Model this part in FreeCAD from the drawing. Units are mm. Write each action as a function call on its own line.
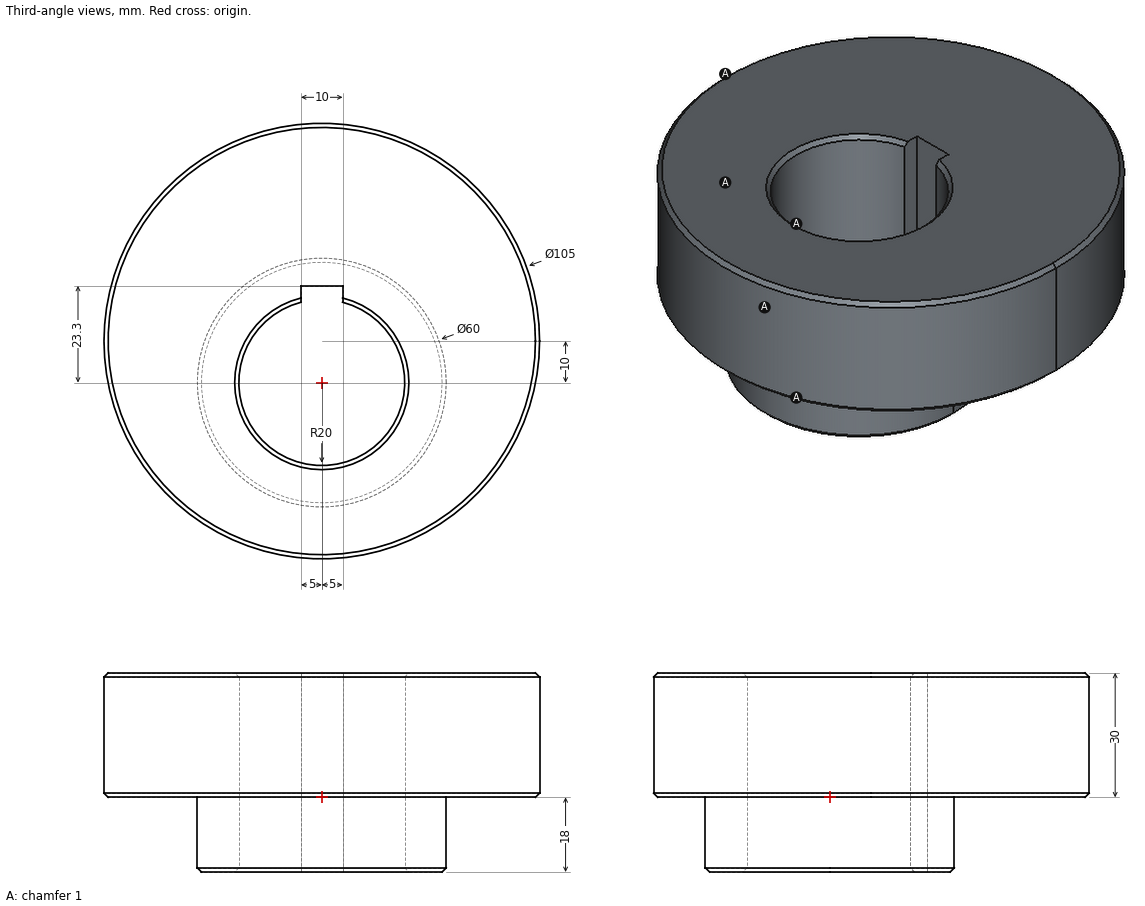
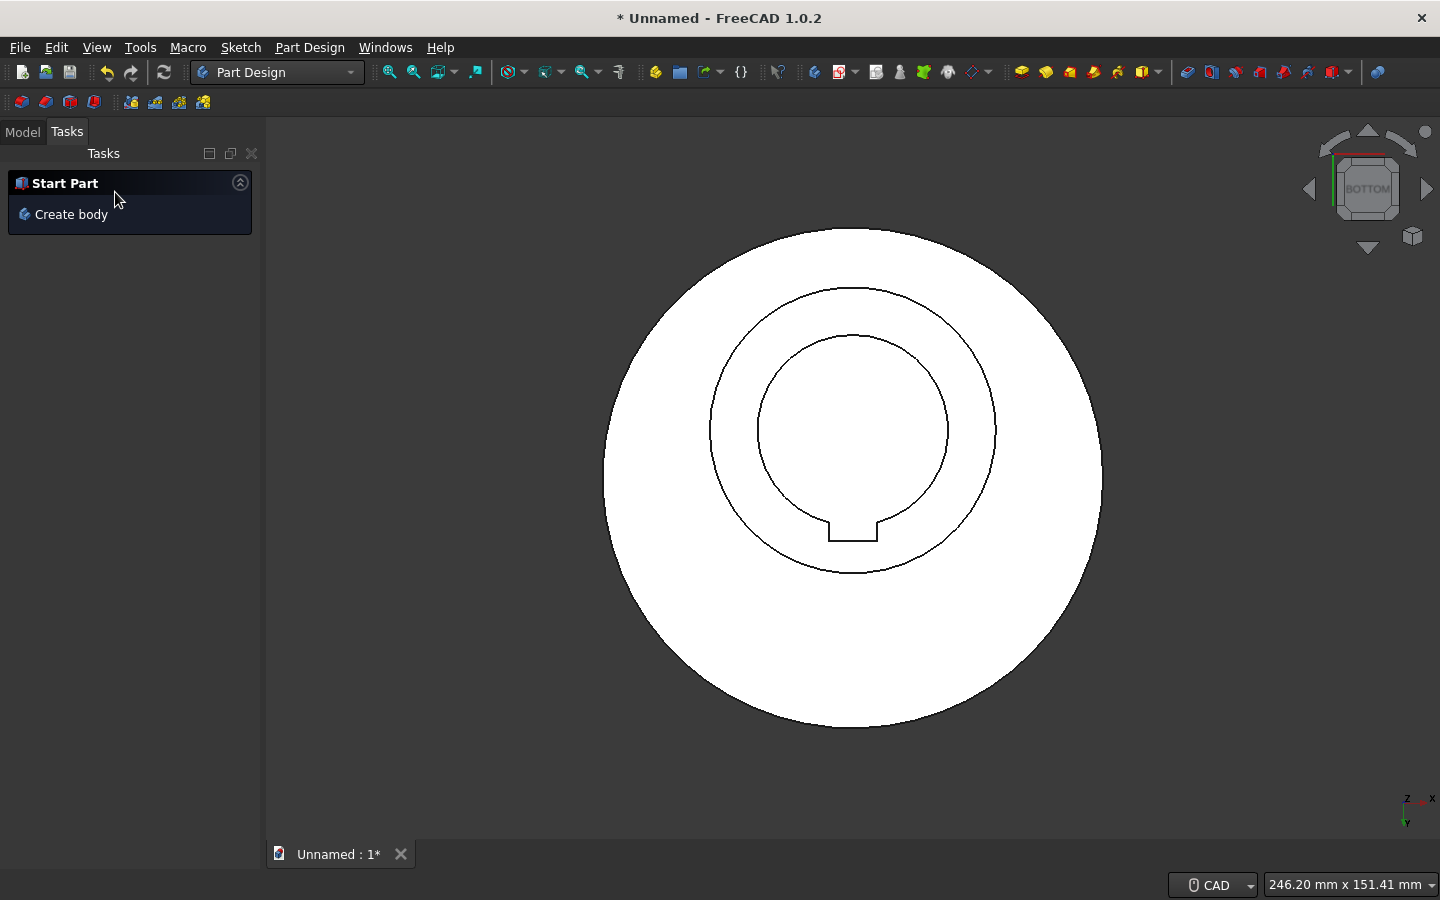
click(840, 72)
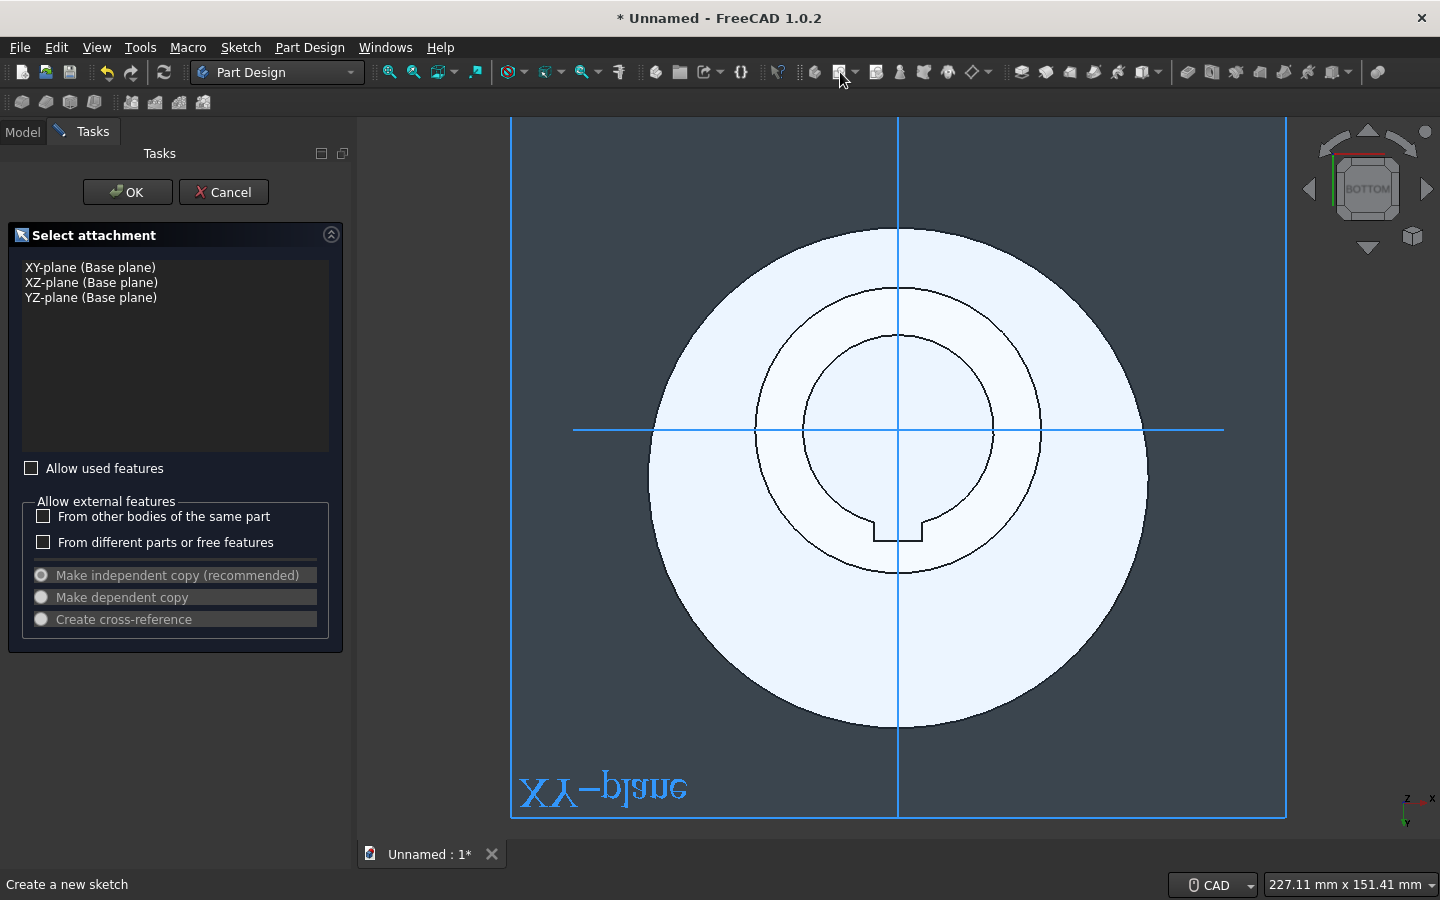
click(82, 268)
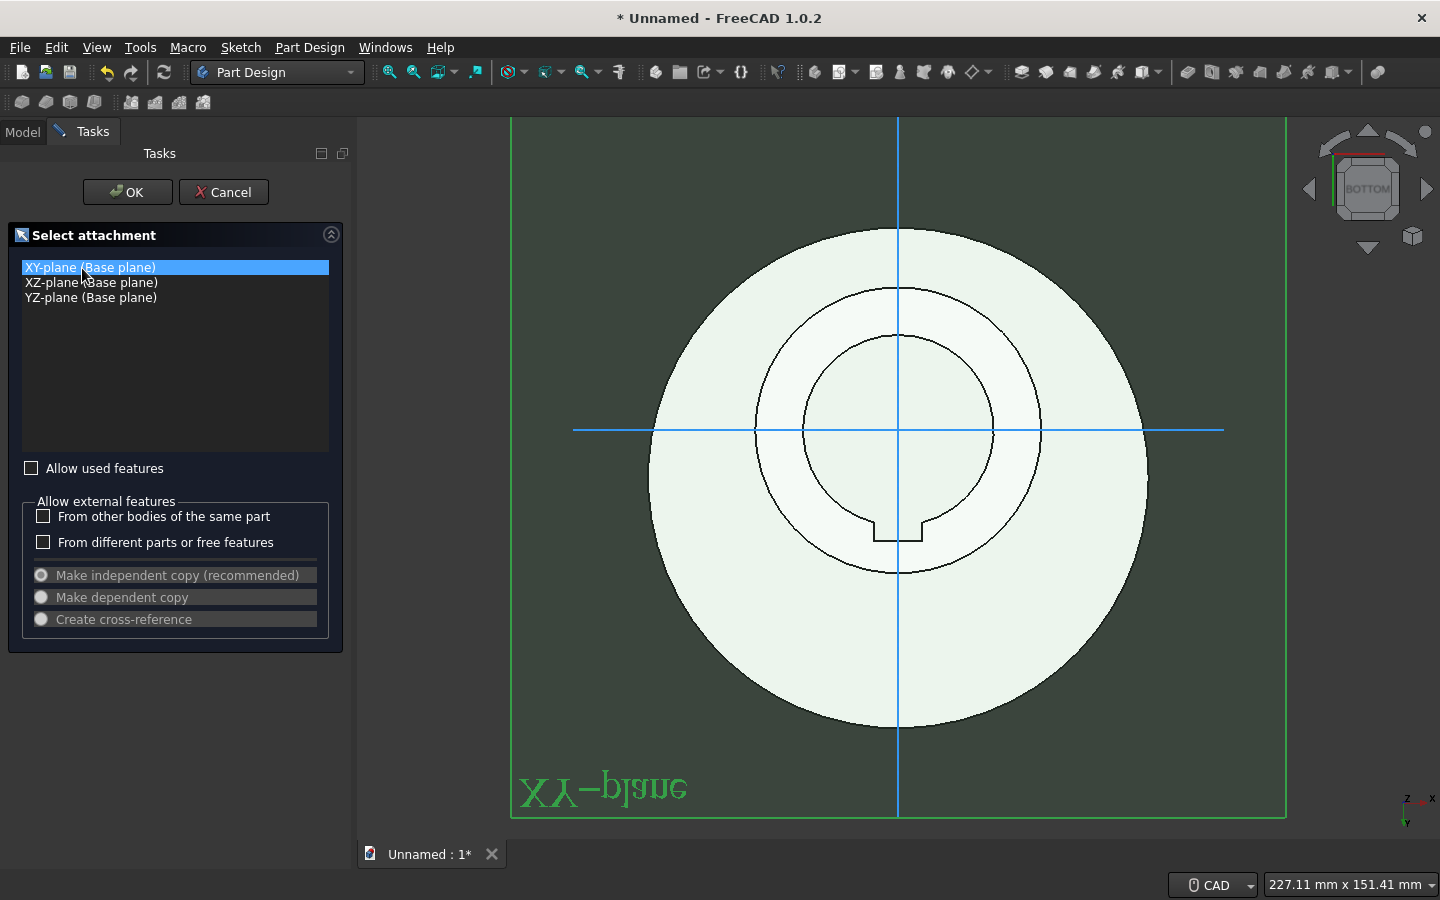
click(128, 192)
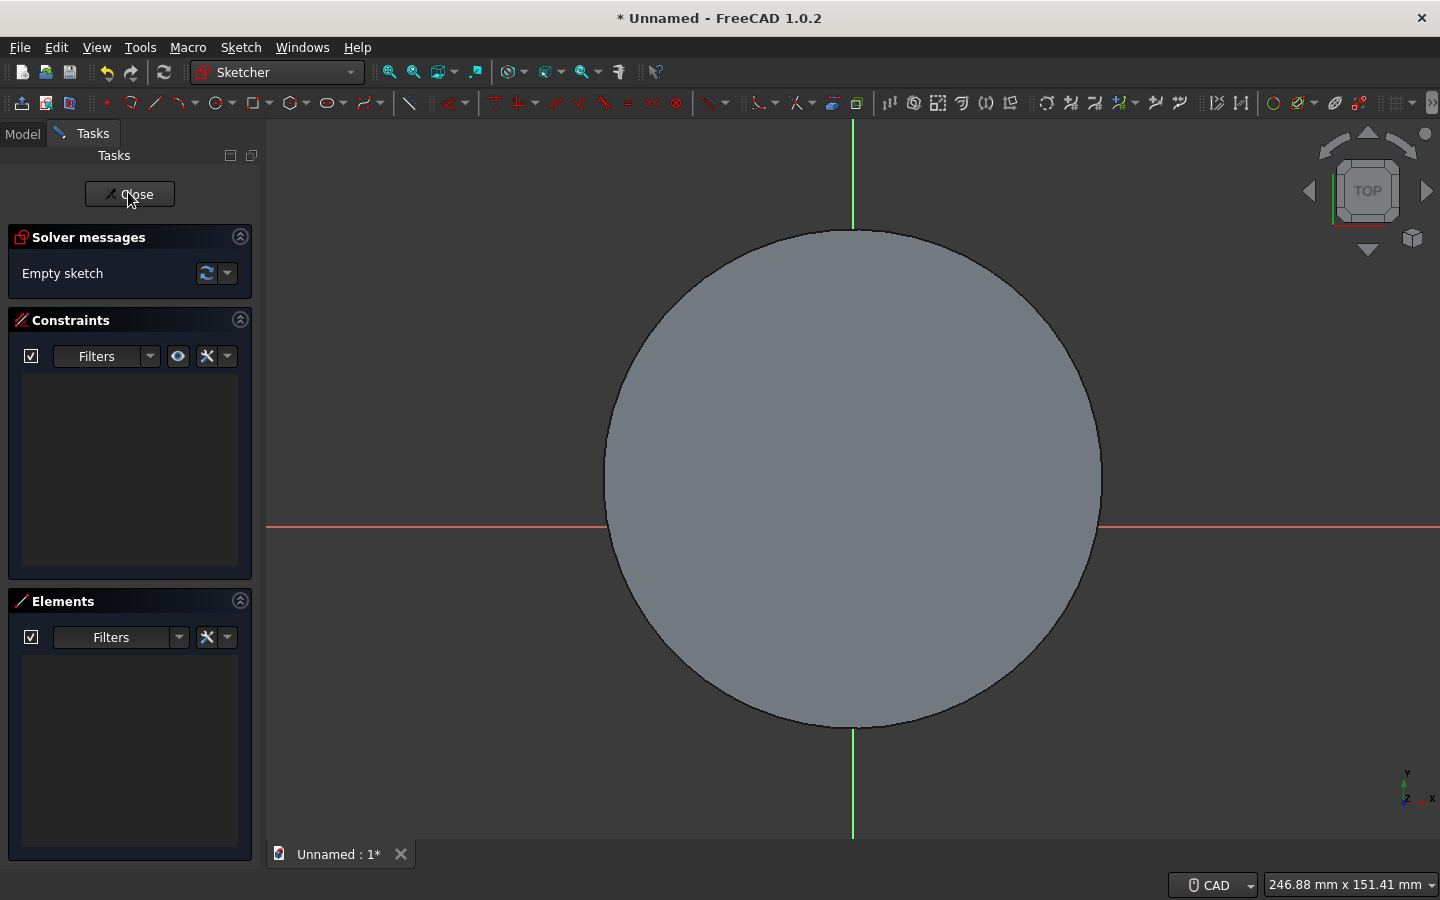
click(70, 104)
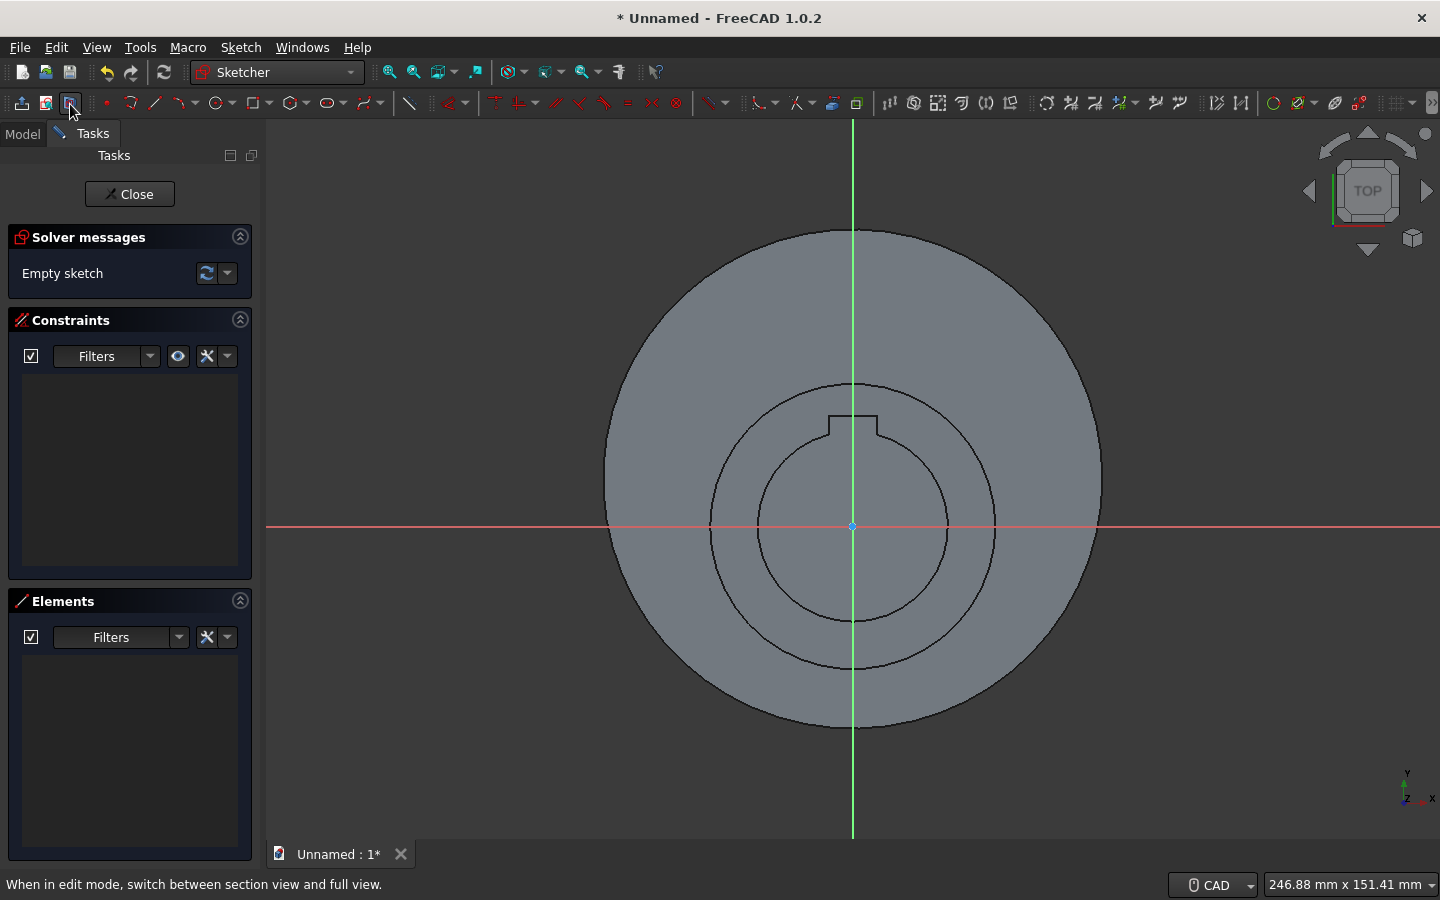
scroll(909, 551, up, 4)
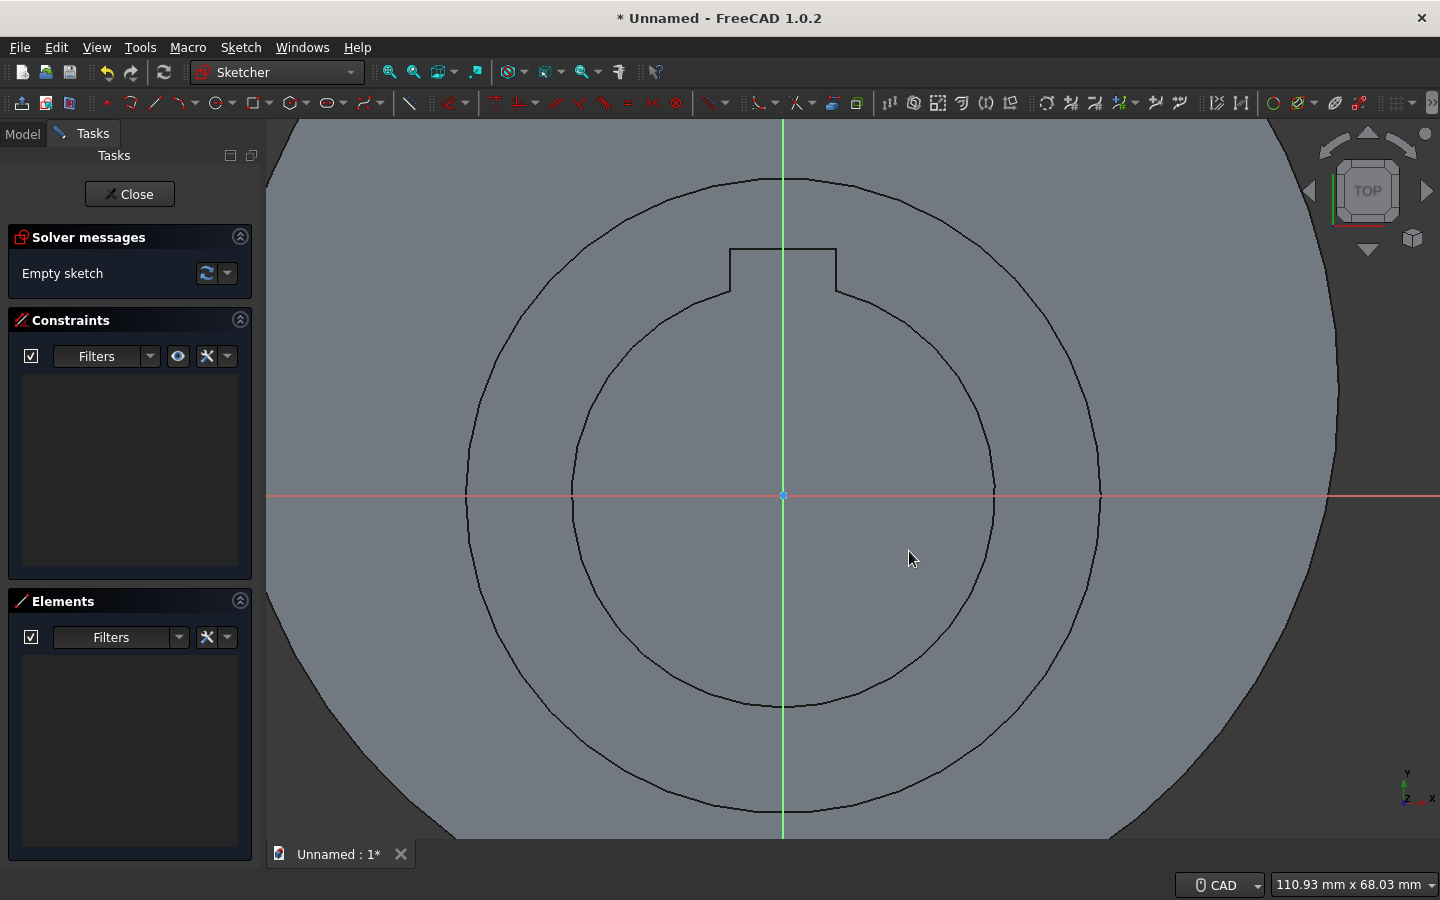
click(132, 104)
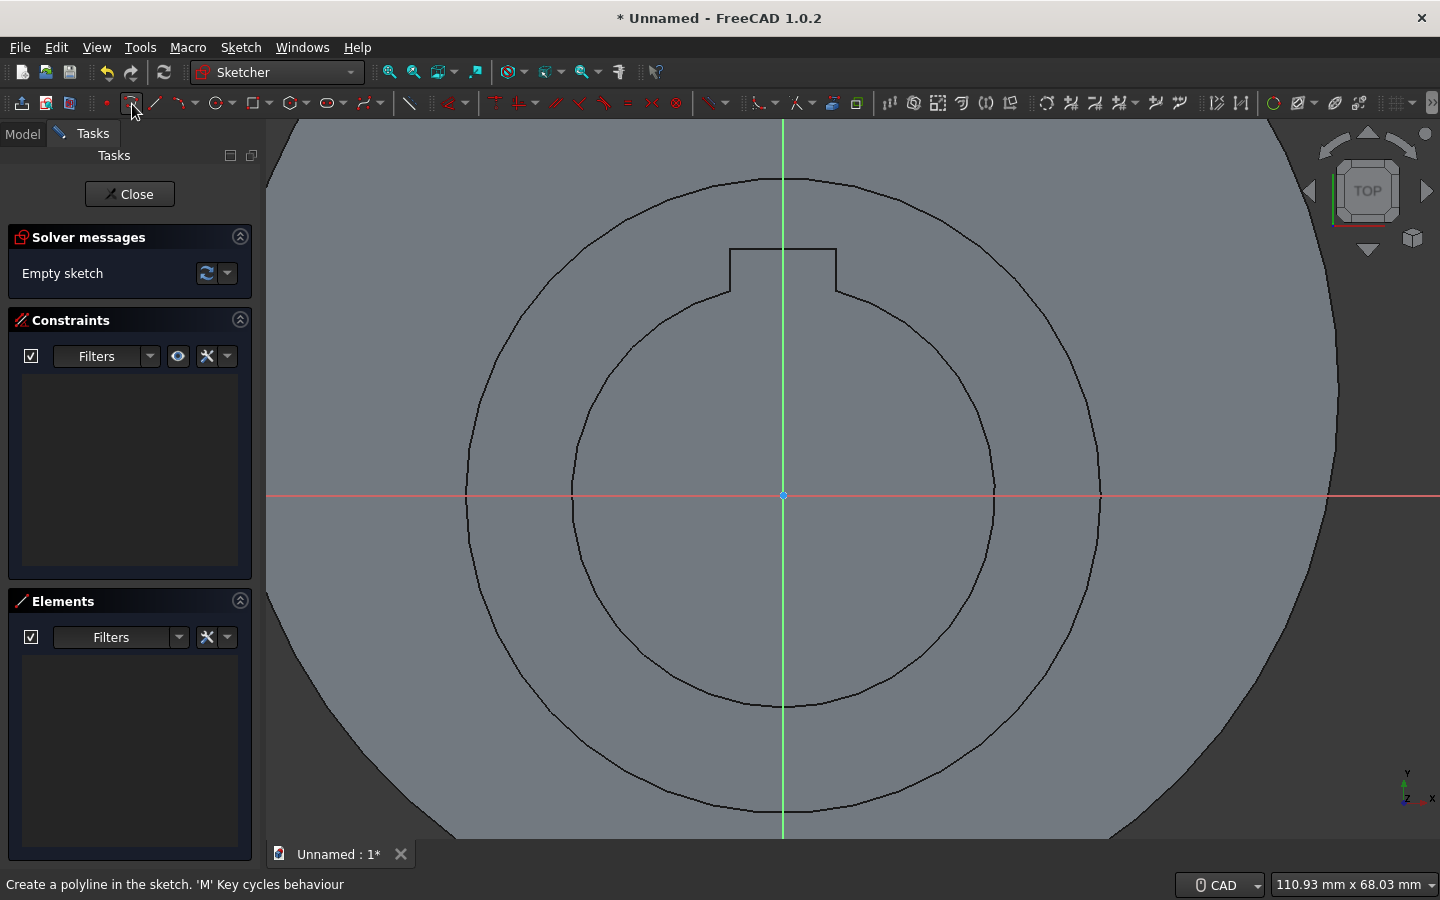
click(836, 291)
click(836, 249)
click(730, 249)
click(730, 291)
right_click(730, 291)